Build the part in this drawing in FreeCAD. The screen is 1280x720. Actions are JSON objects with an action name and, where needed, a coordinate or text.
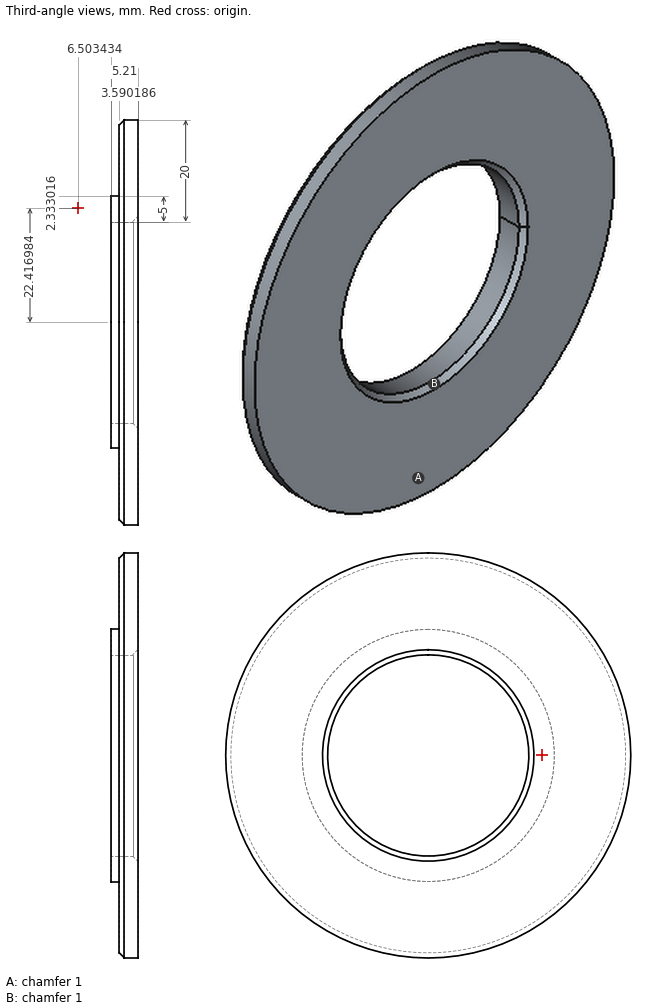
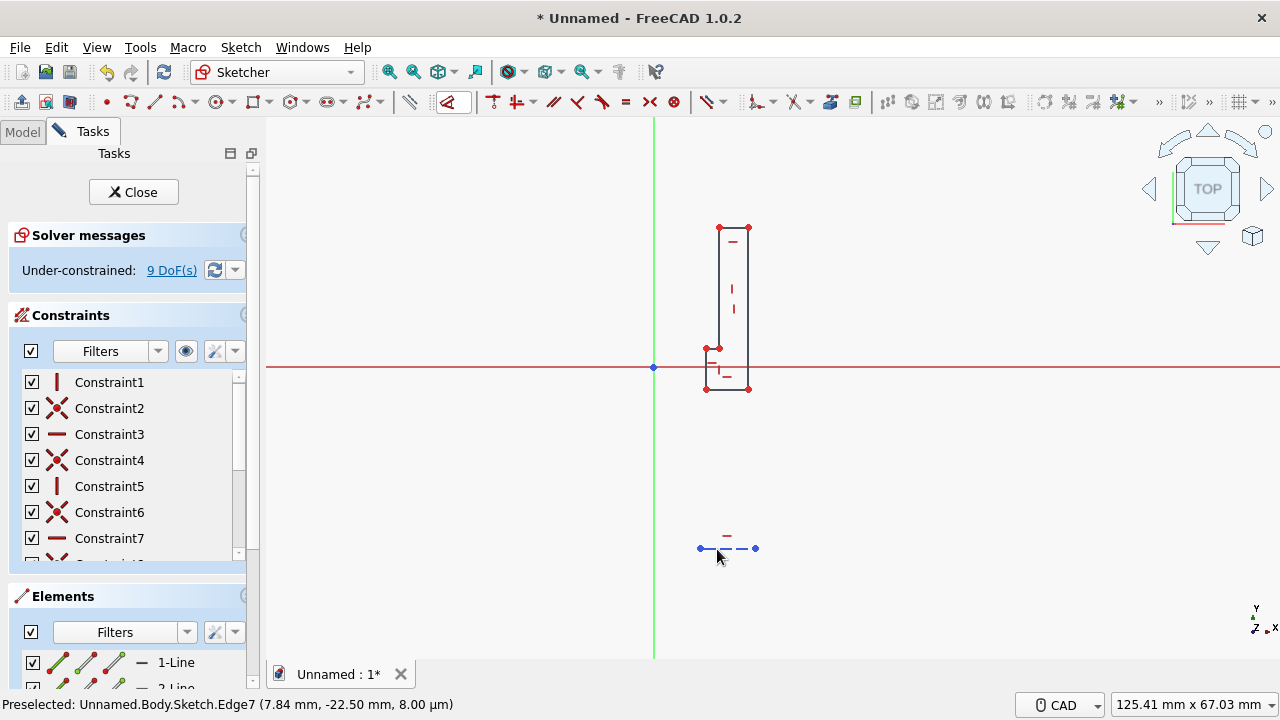
{"action": "scroll", "coordinate": [706, 378], "scroll_direction": "up", "scroll_amount": 2}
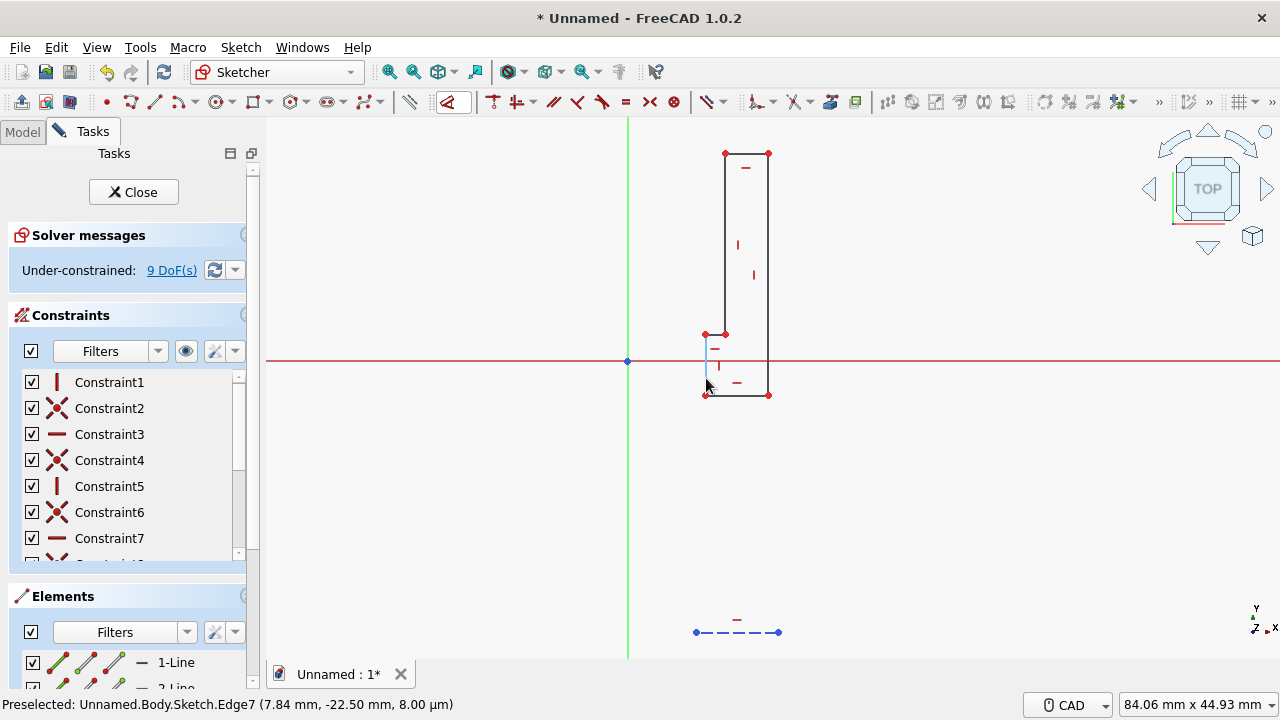
{"action": "left_click", "coordinate": [706, 377]}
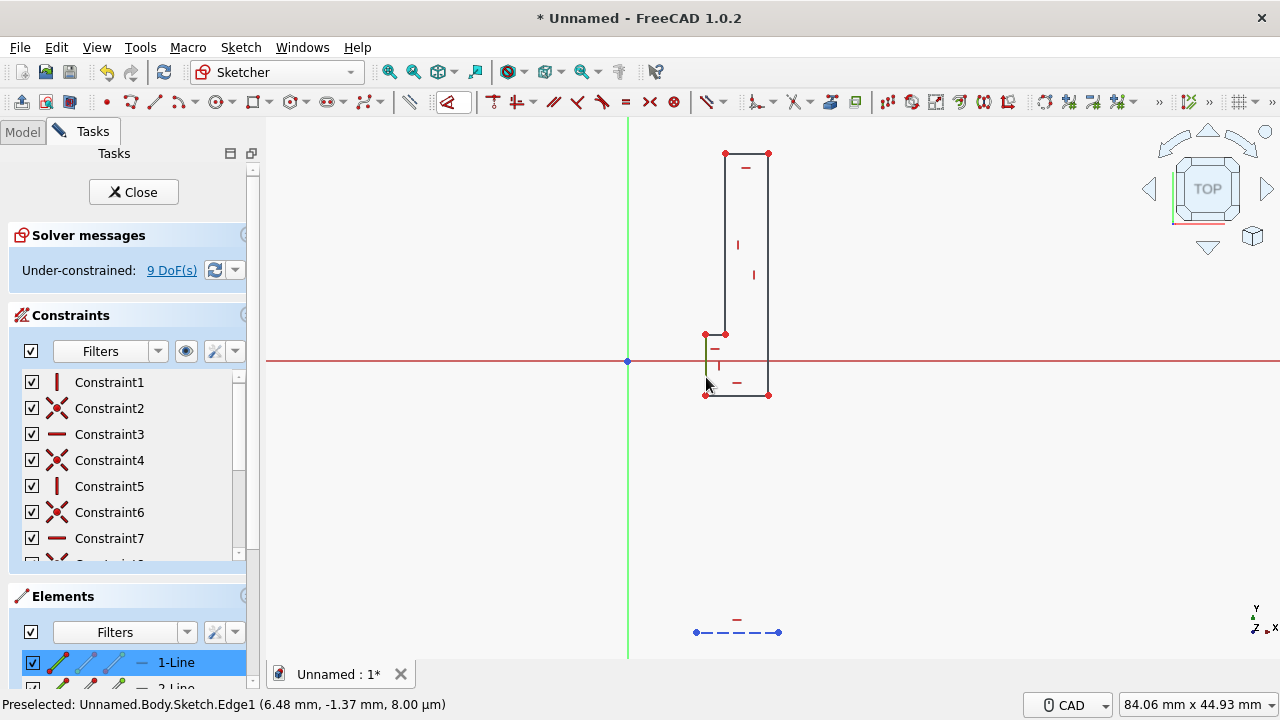
{"action": "key", "text": "i"}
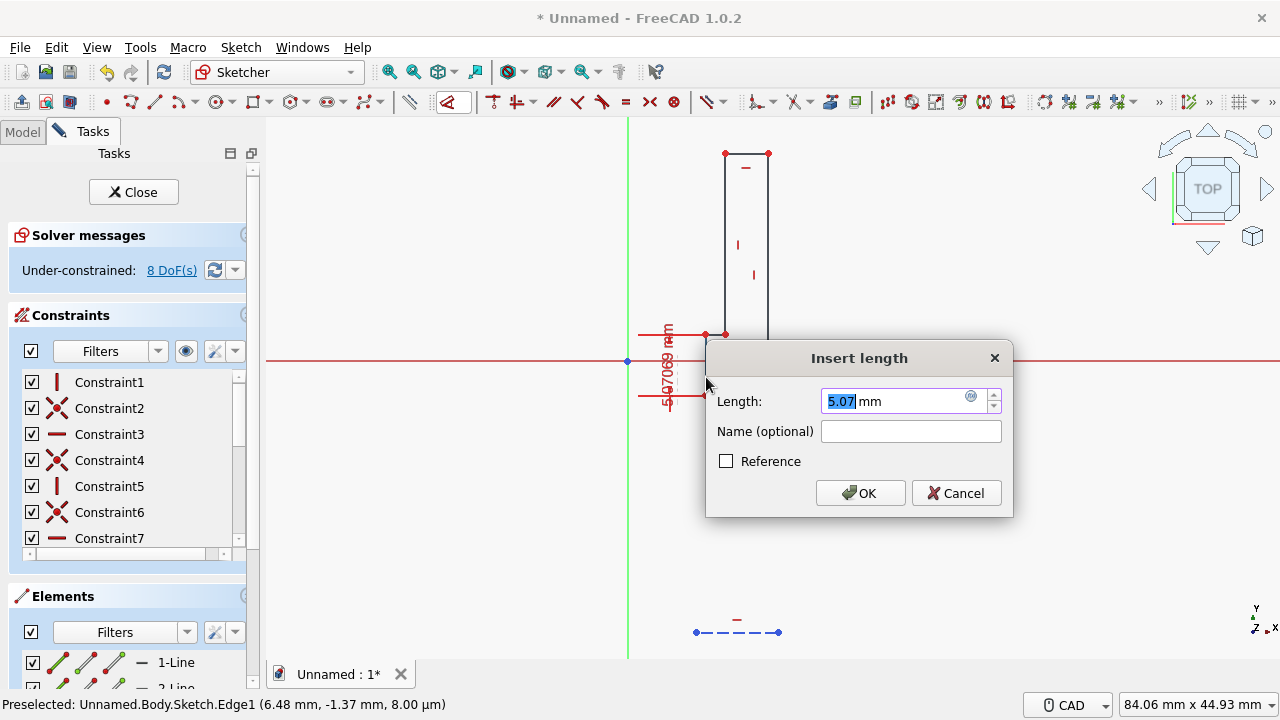
{"action": "type", "text": "5"}
{"action": "key", "text": "Return"}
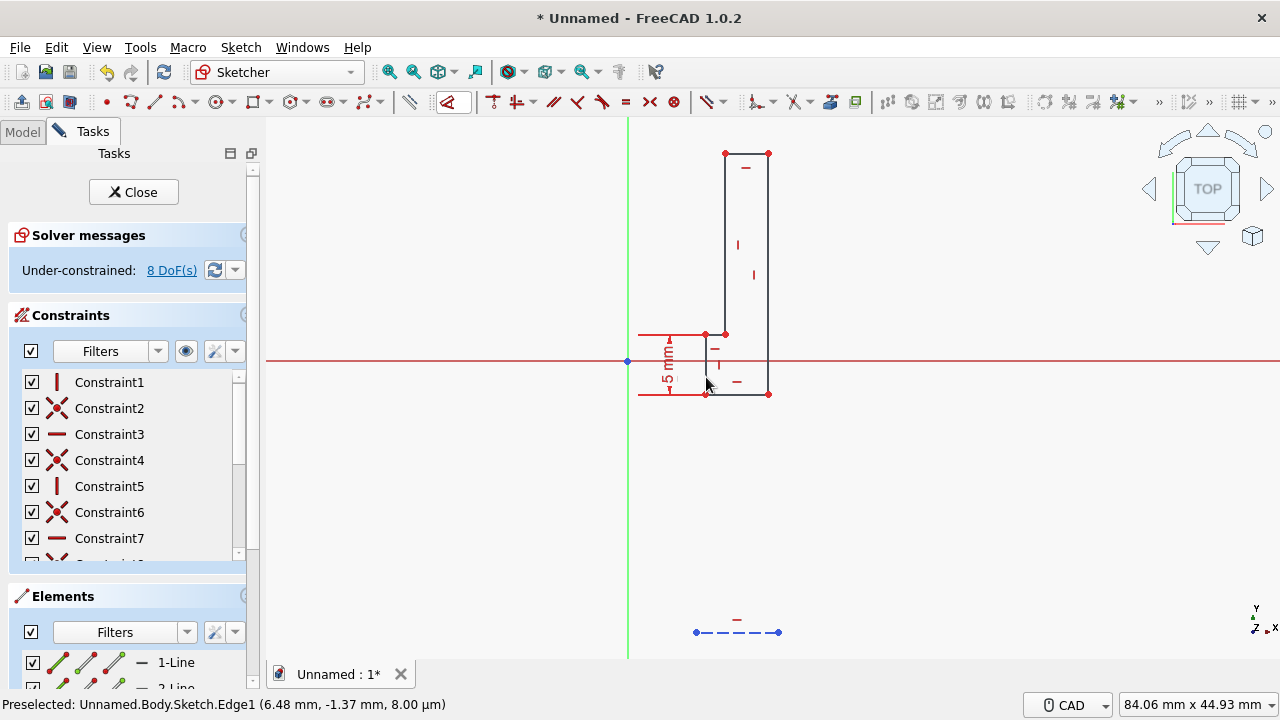
{"action": "left_click", "coordinate": [768, 323]}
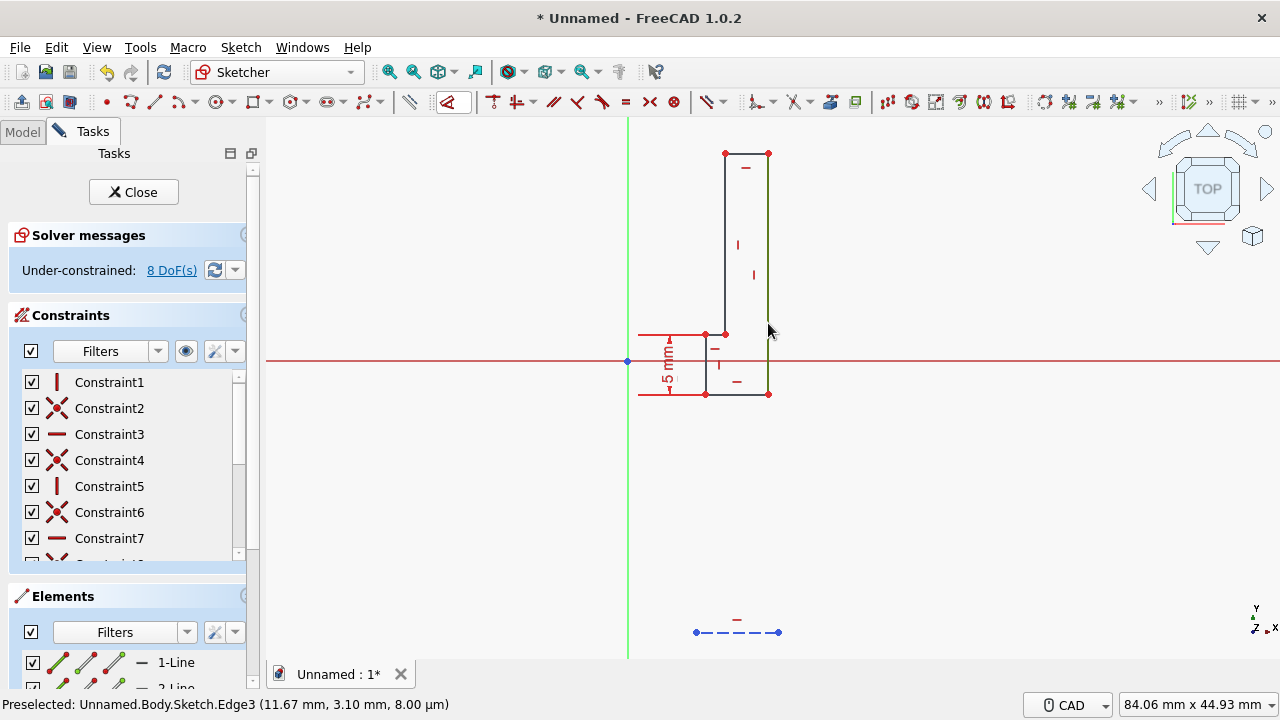
{"action": "key", "text": "i"}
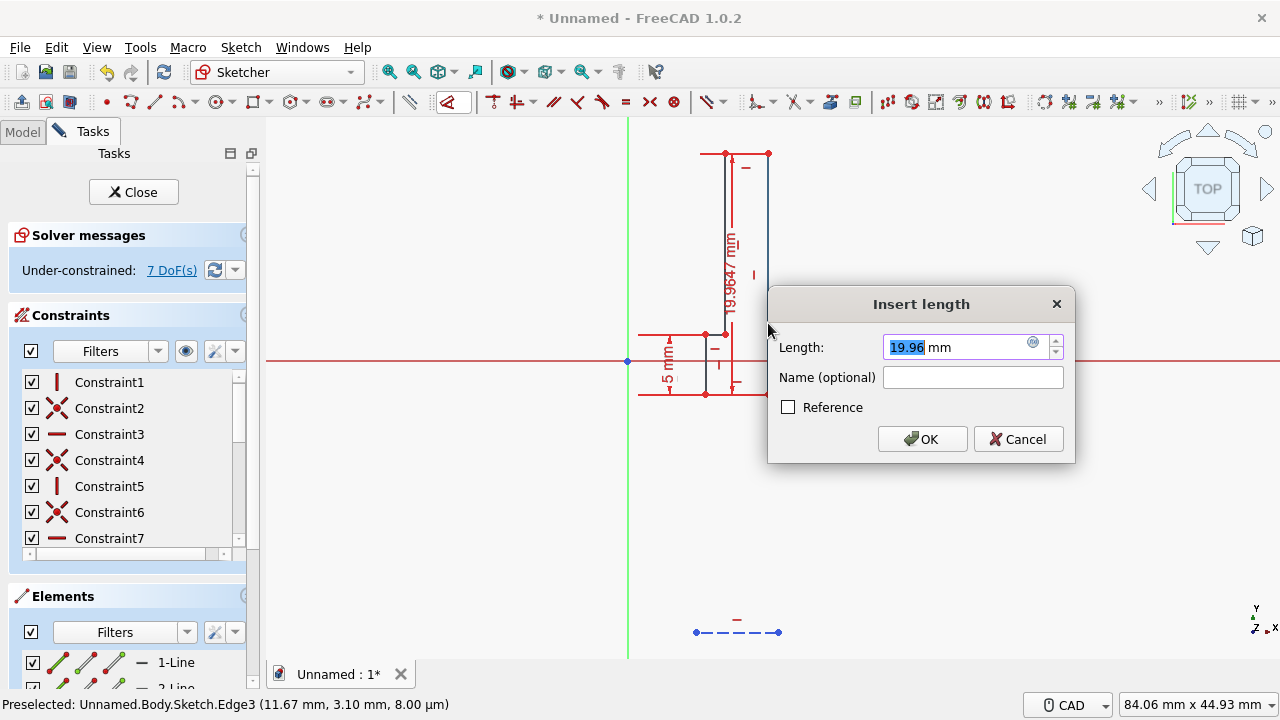
{"action": "type", "text": "20"}
{"action": "key", "text": "Return"}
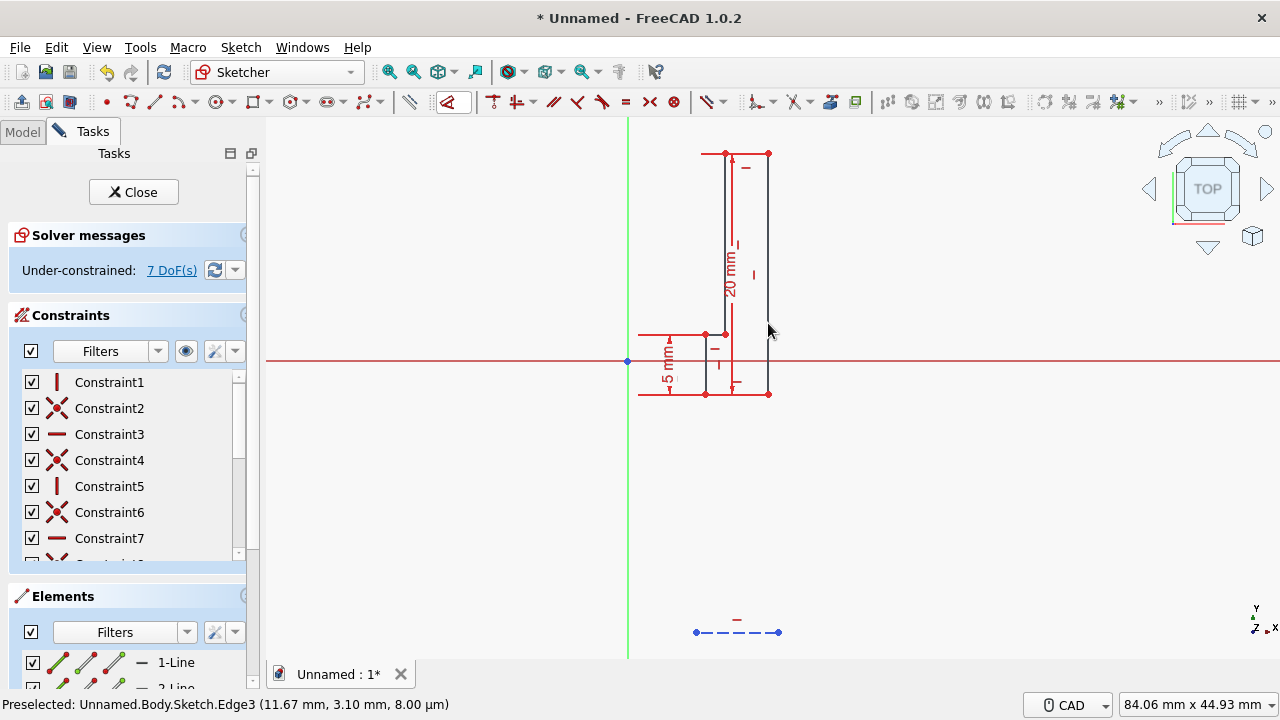
{"action": "left_click", "coordinate": [725, 395]}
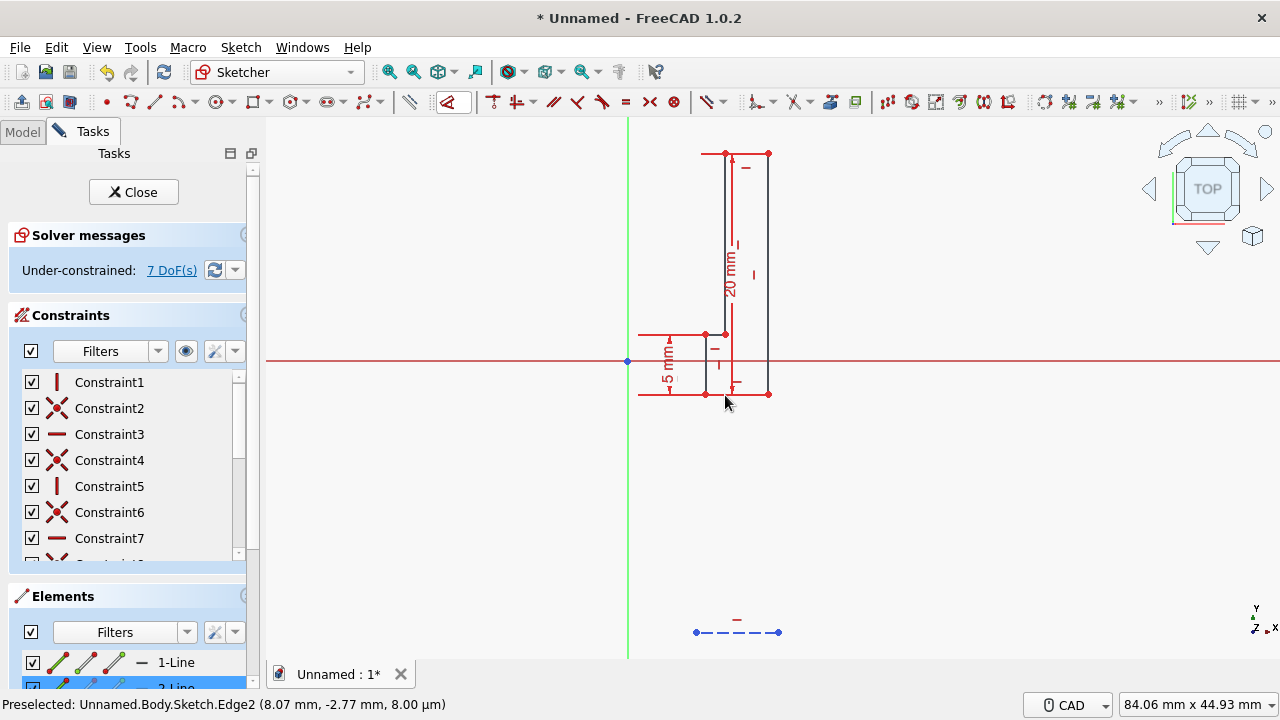
{"action": "key", "text": "l"}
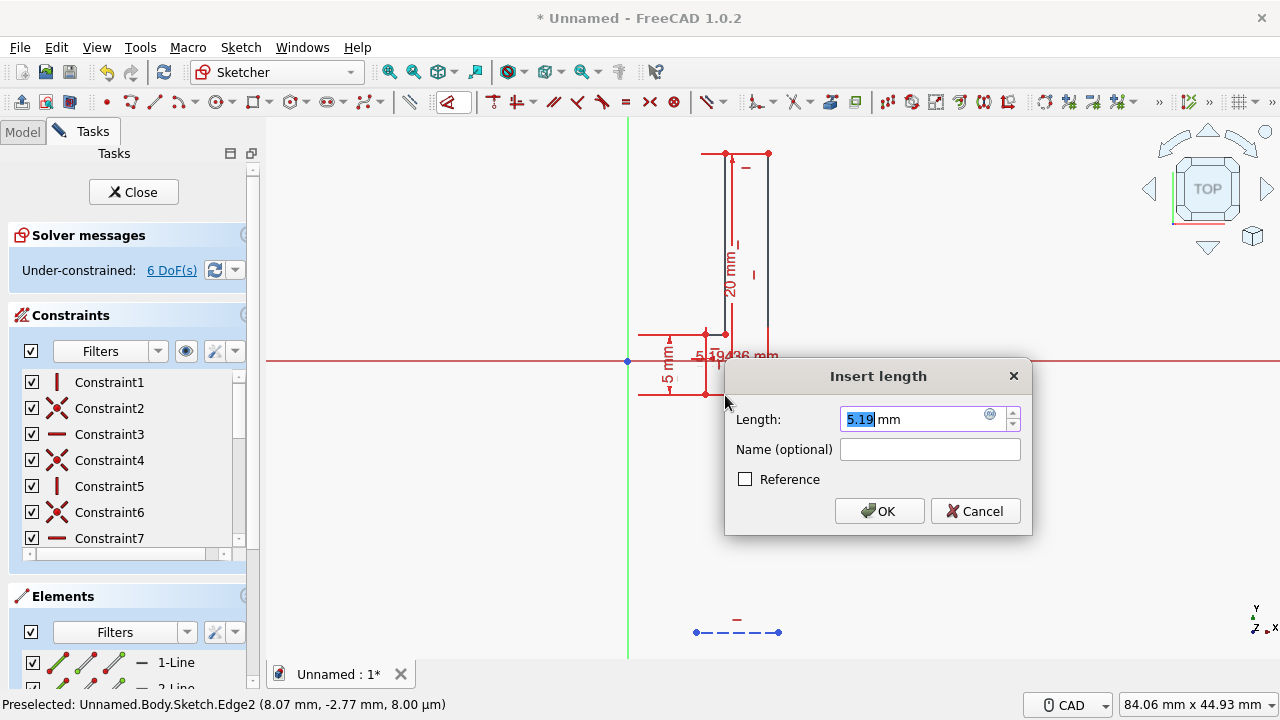
{"action": "type", "text": "5.21"}
{"action": "key", "text": "Return"}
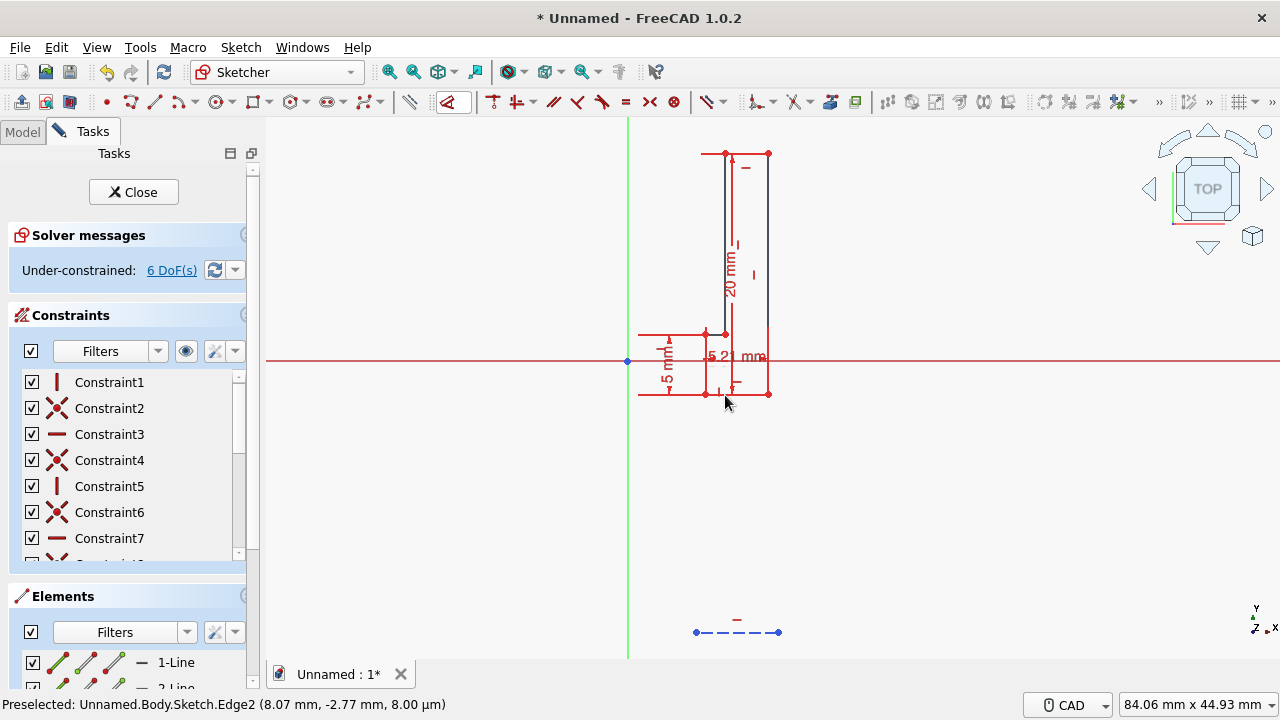
{"action": "left_click", "coordinate": [755, 154]}